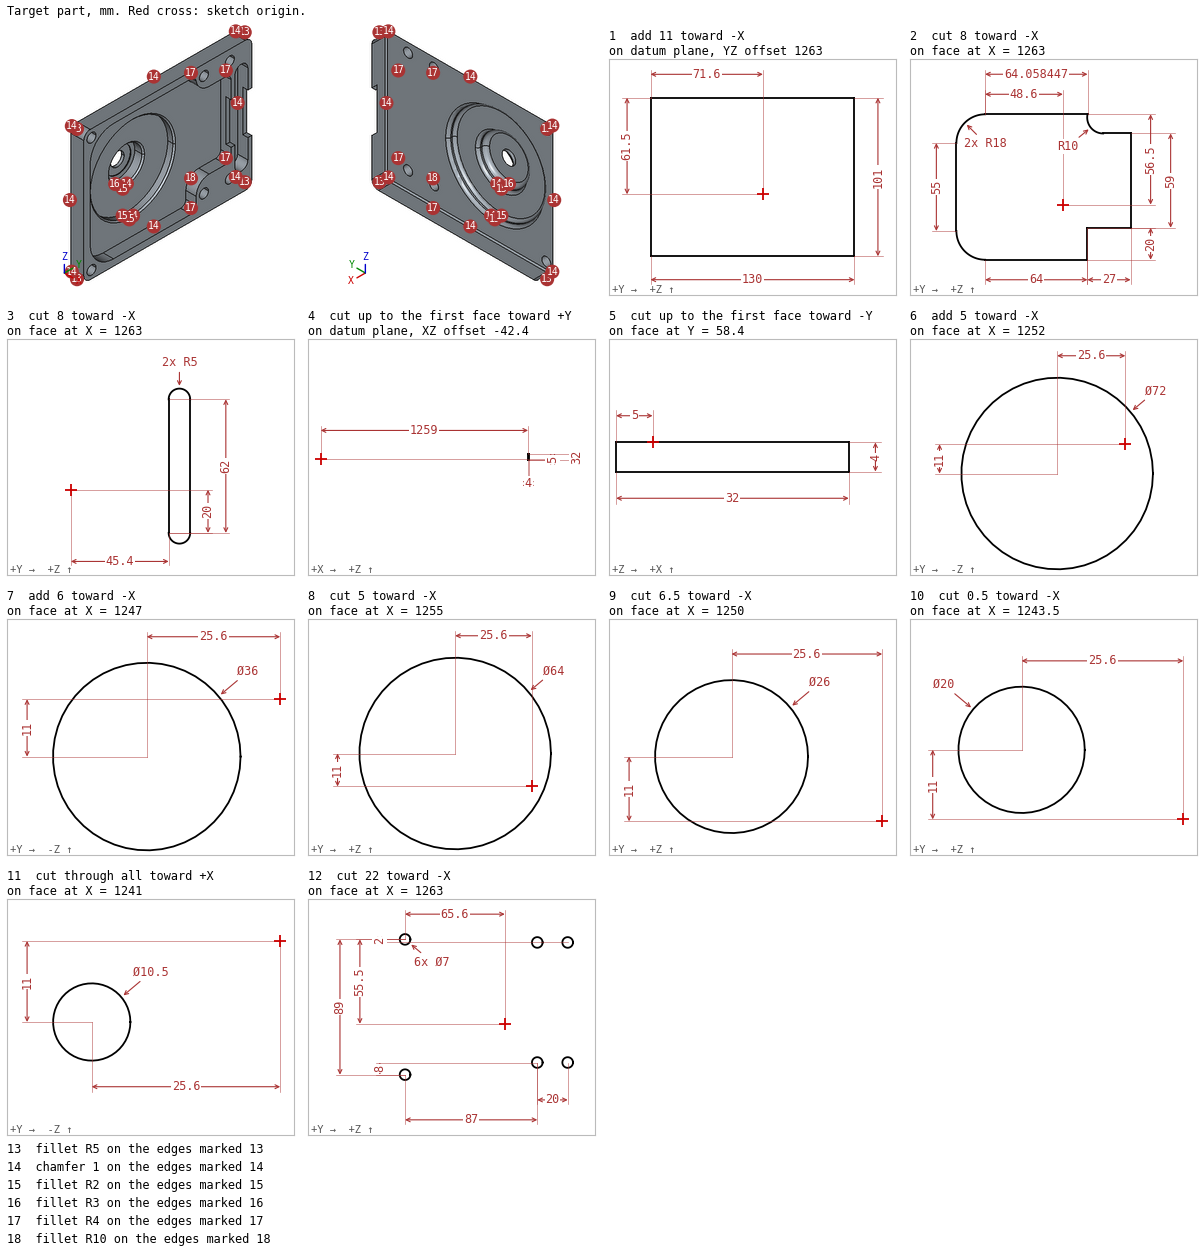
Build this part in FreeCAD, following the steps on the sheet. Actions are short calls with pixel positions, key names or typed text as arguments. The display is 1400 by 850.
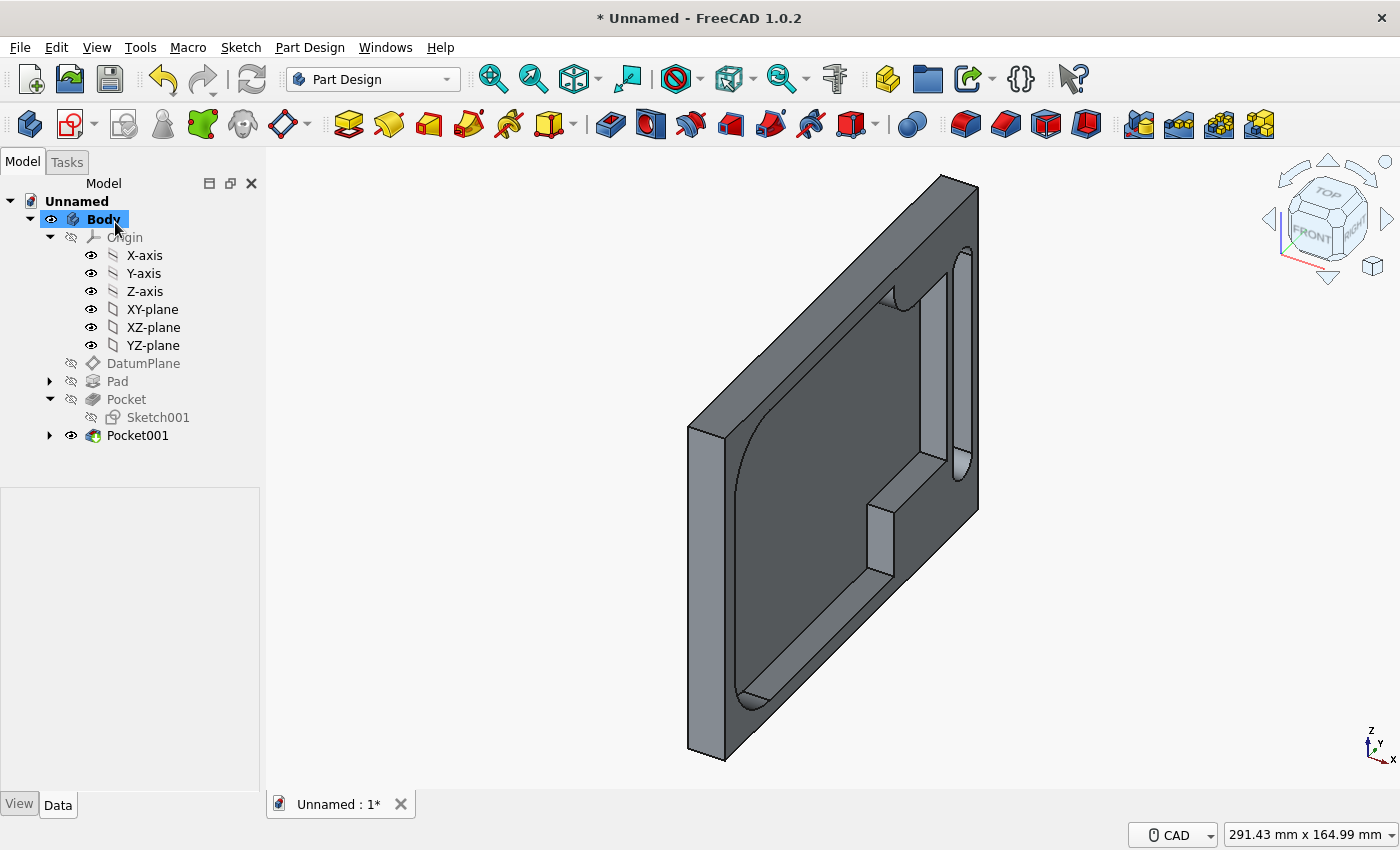
click(136, 327)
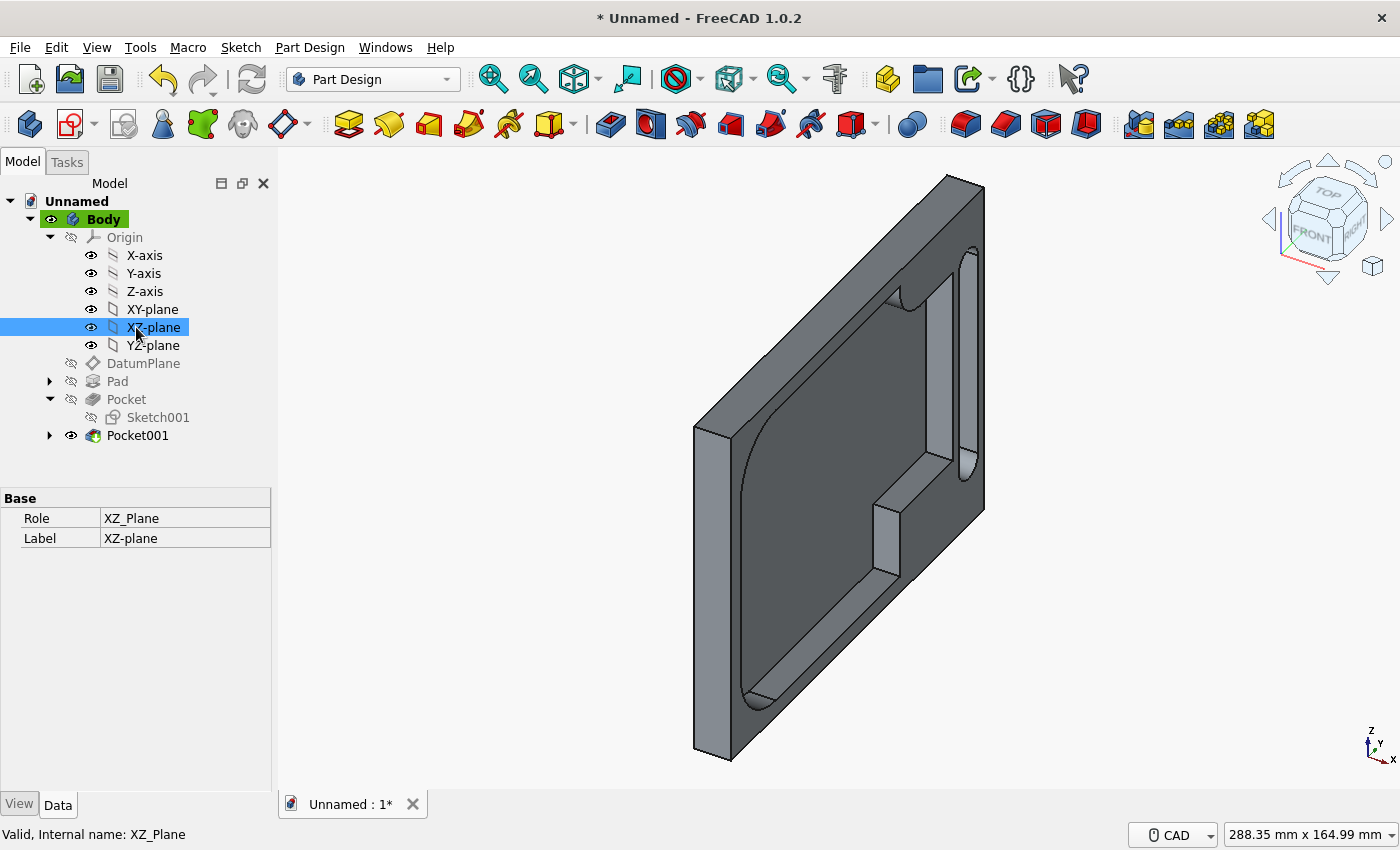
click(284, 124)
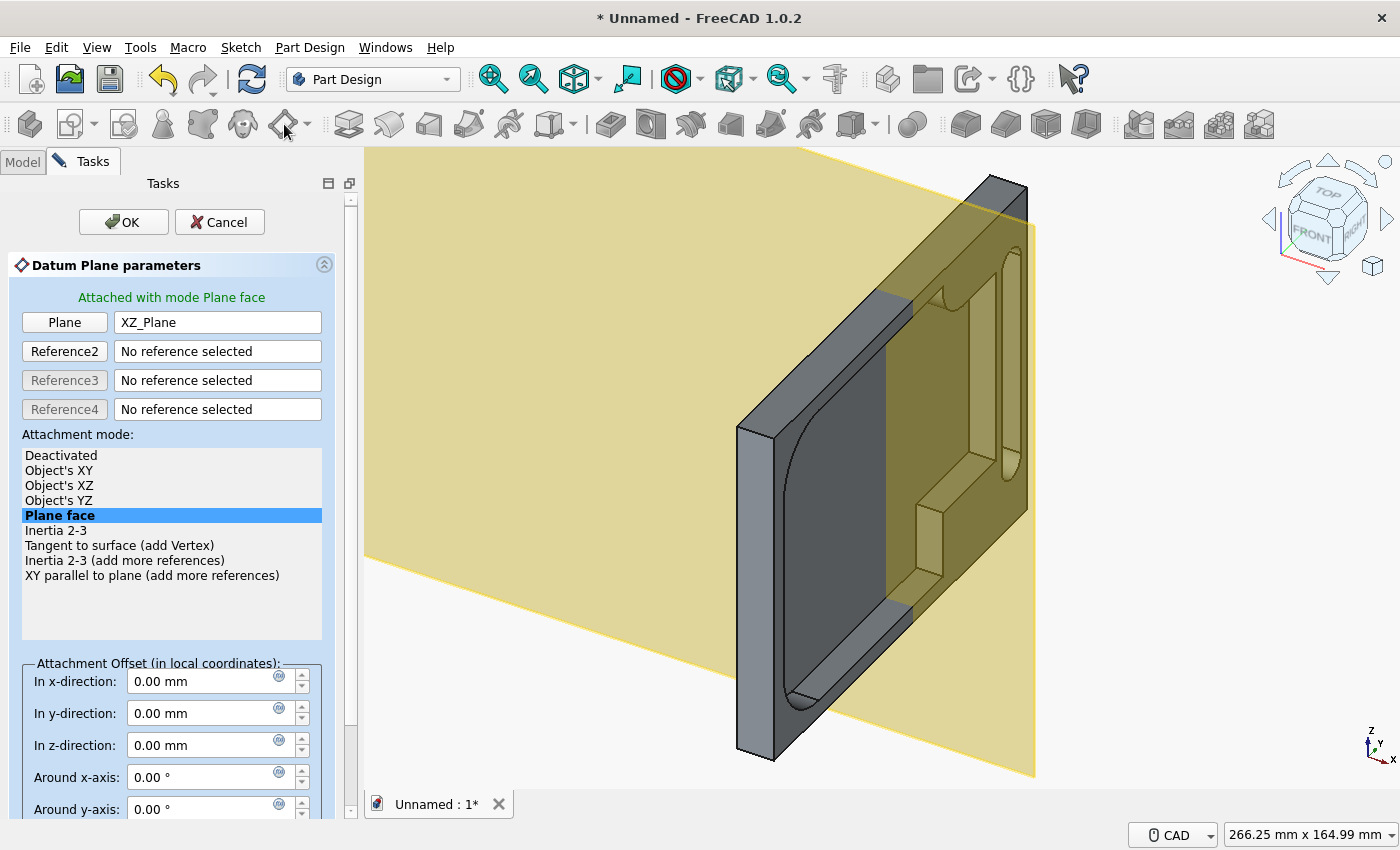
triple_click(210, 745)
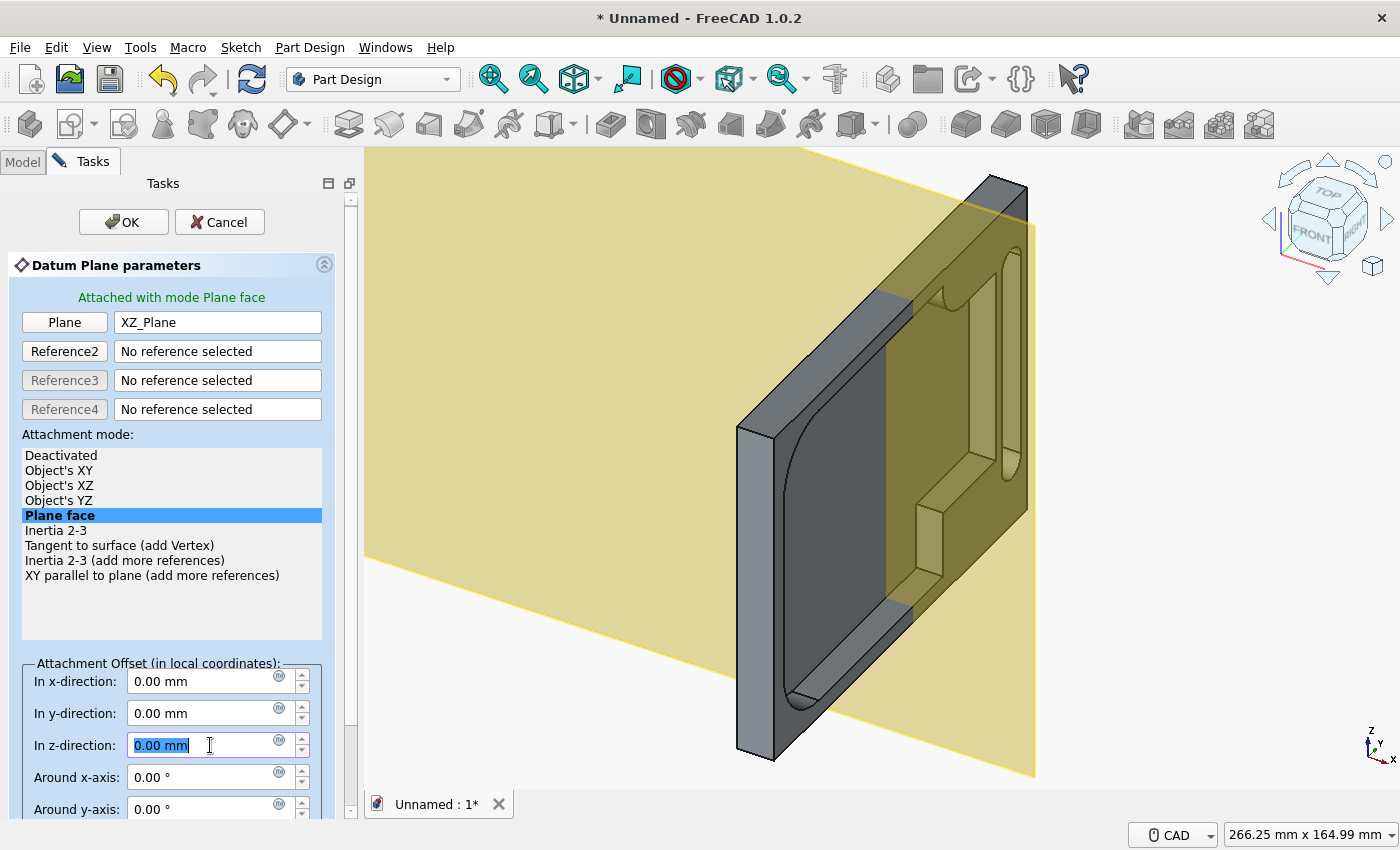
text(-42.4)
key(Tab)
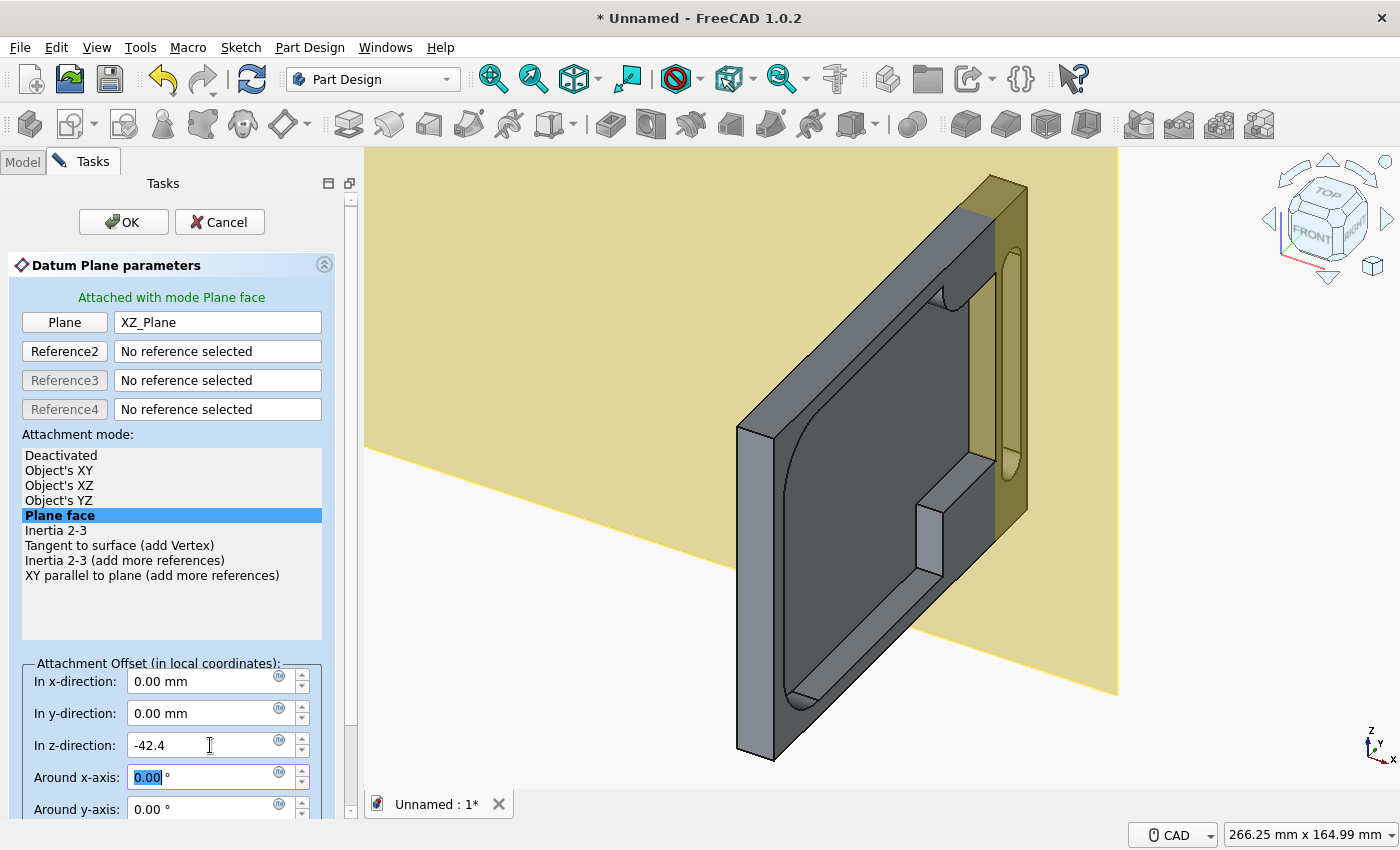
click(124, 222)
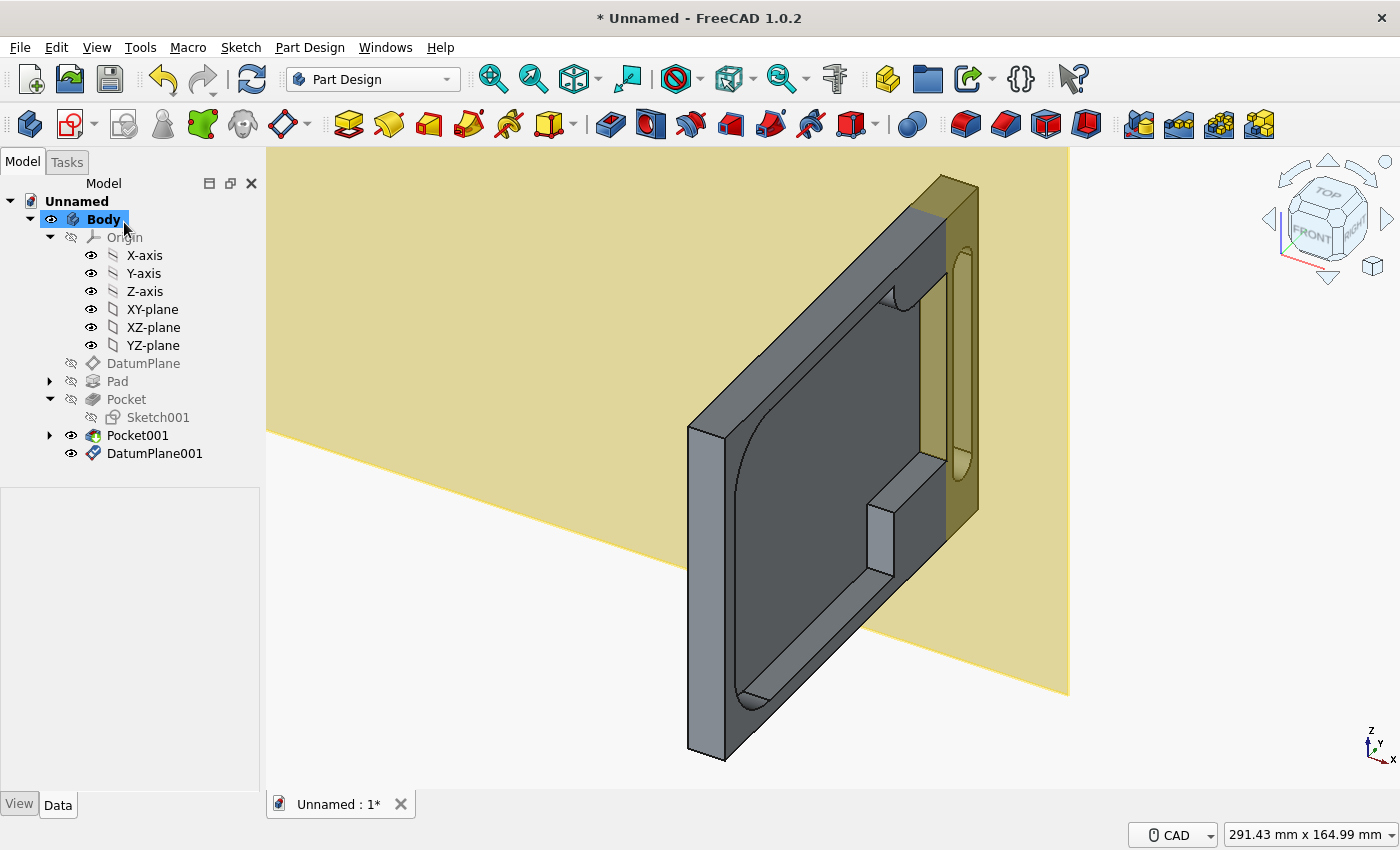
click(116, 453)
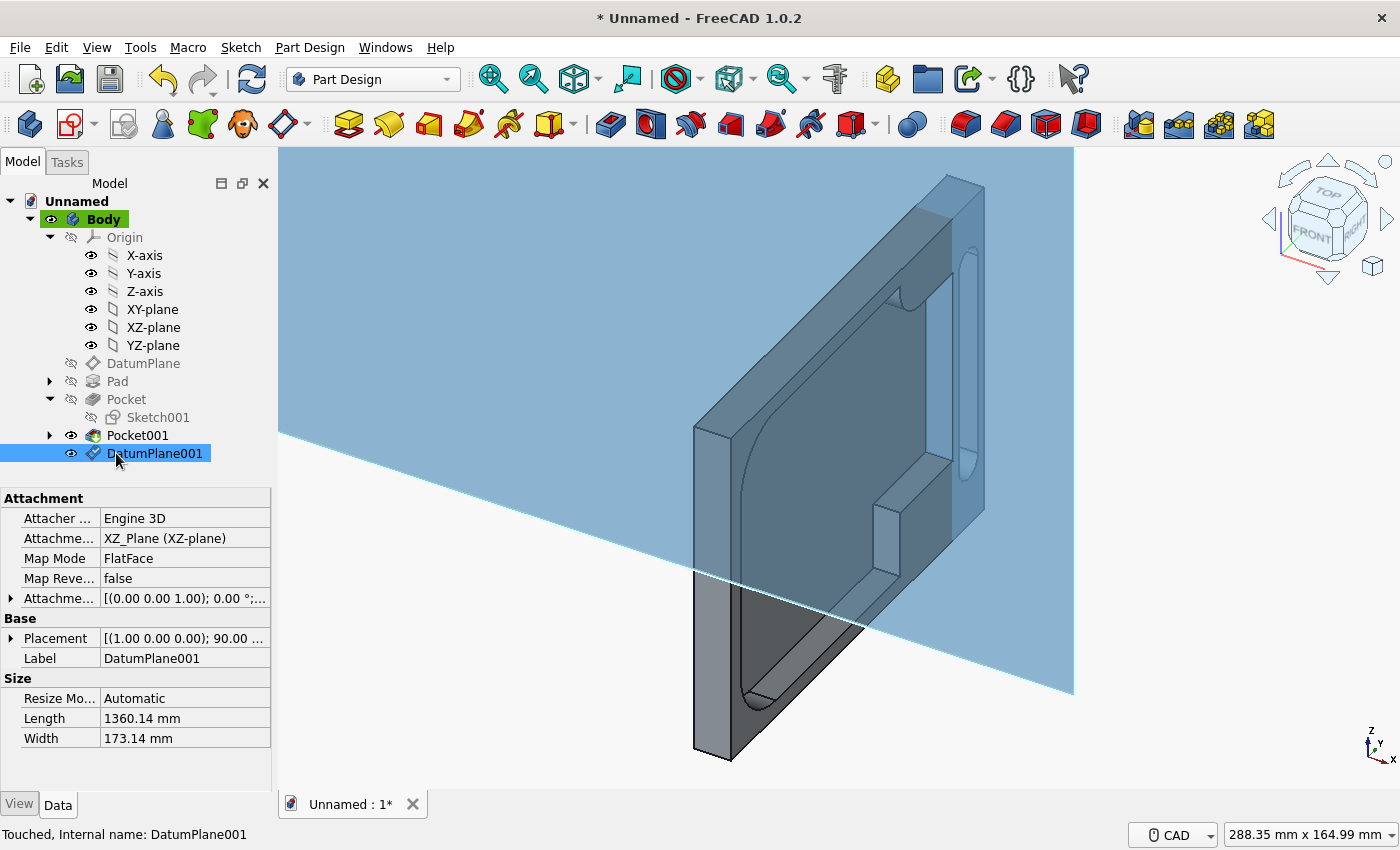
click(70, 124)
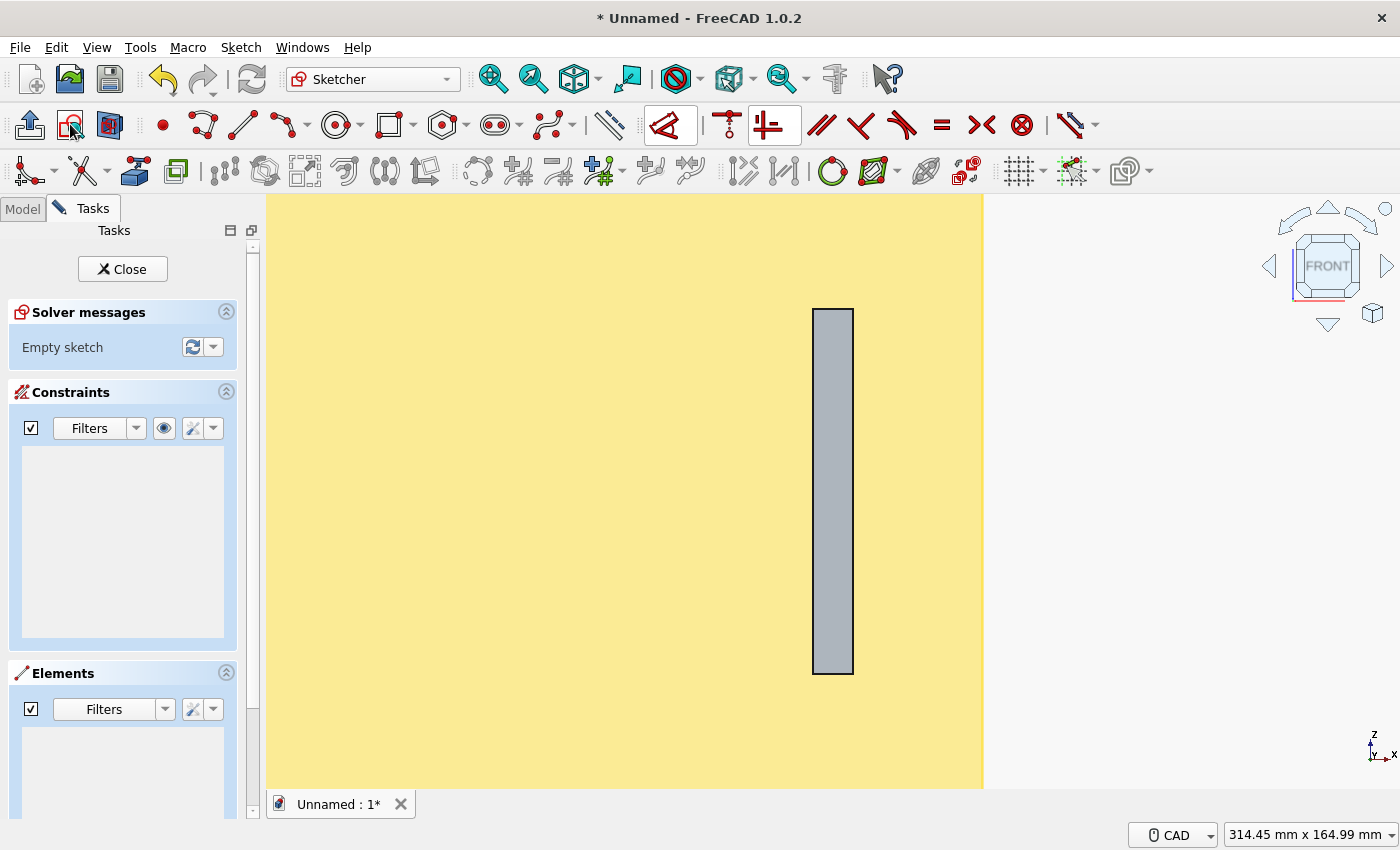
key(q)
key(s)